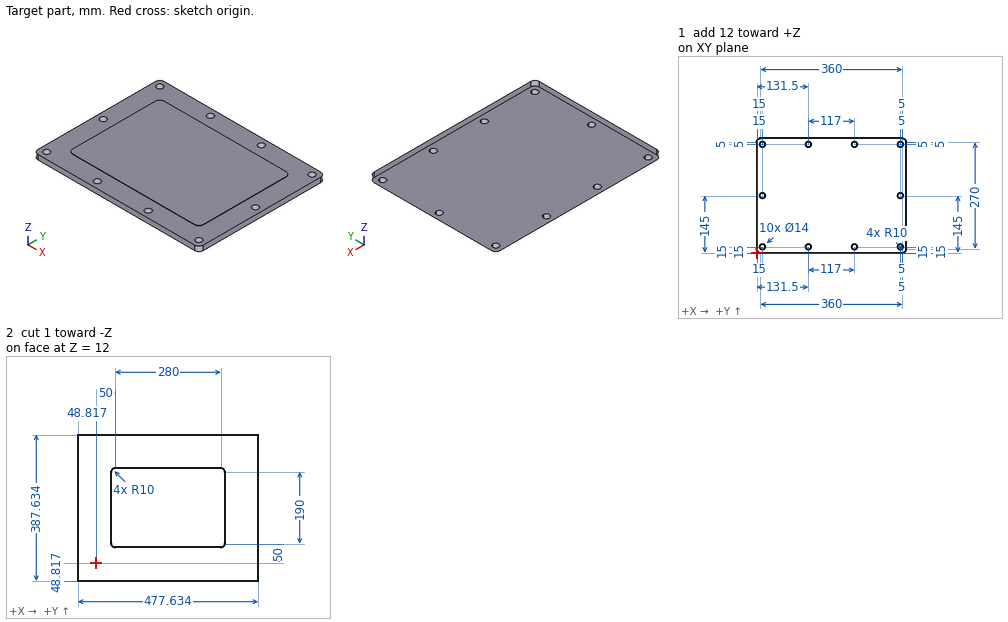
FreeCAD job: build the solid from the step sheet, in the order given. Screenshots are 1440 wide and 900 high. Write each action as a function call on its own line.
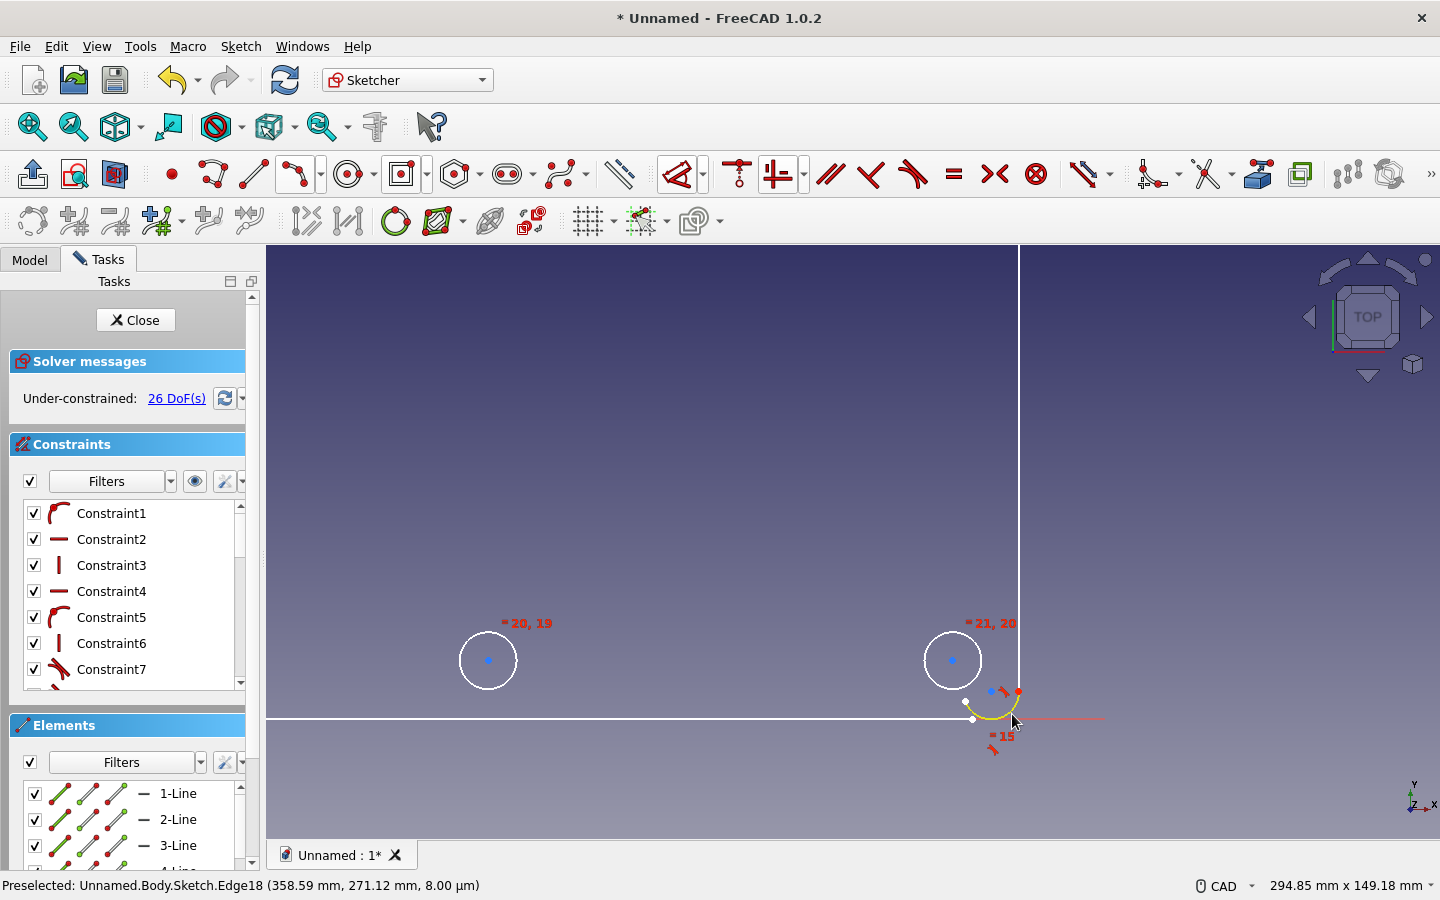
click(1010, 712)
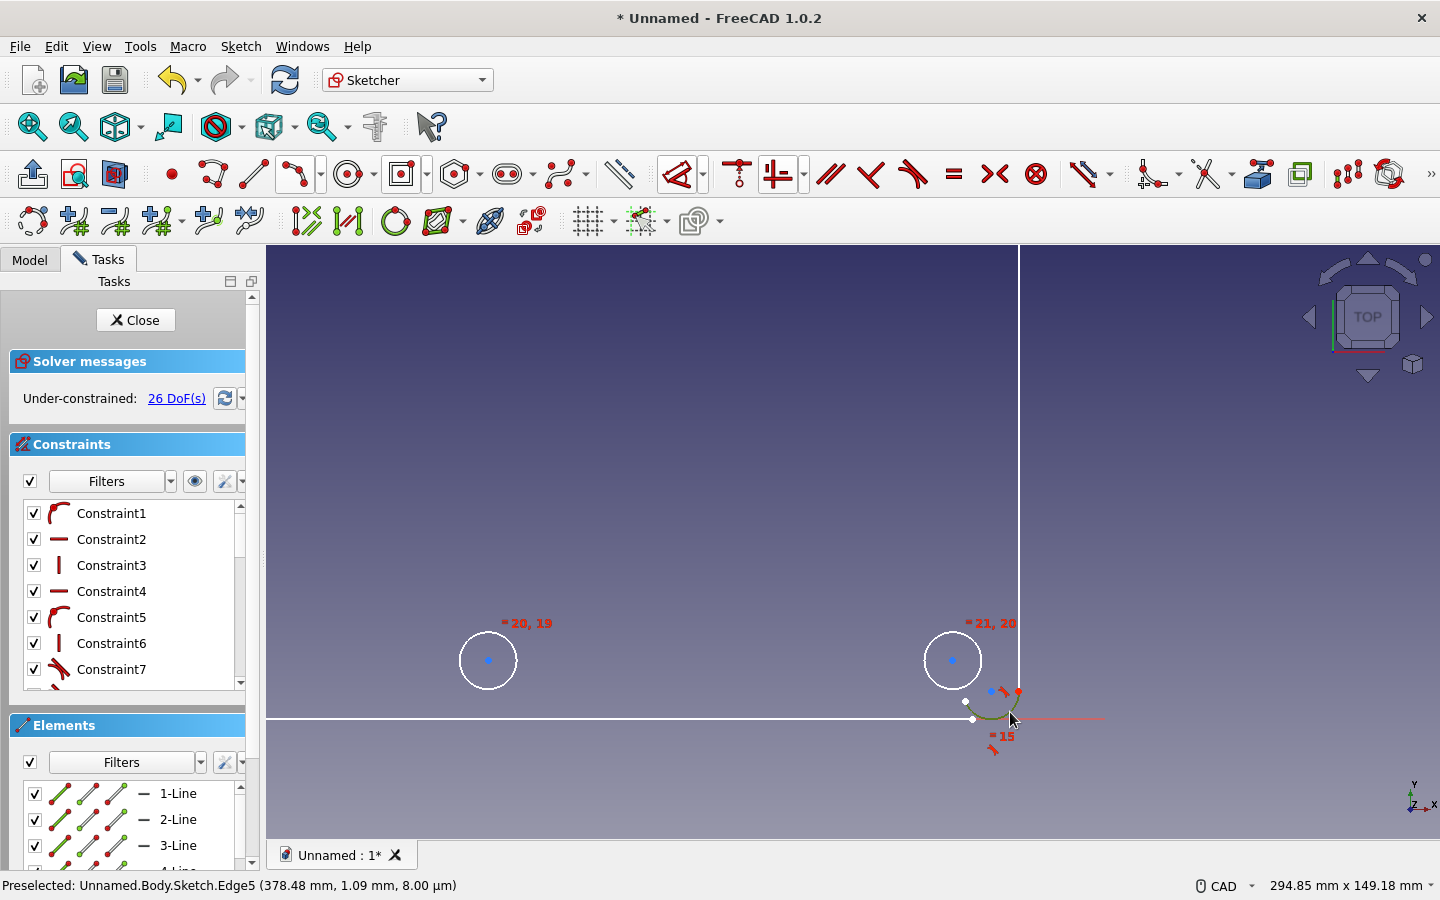
click(702, 174)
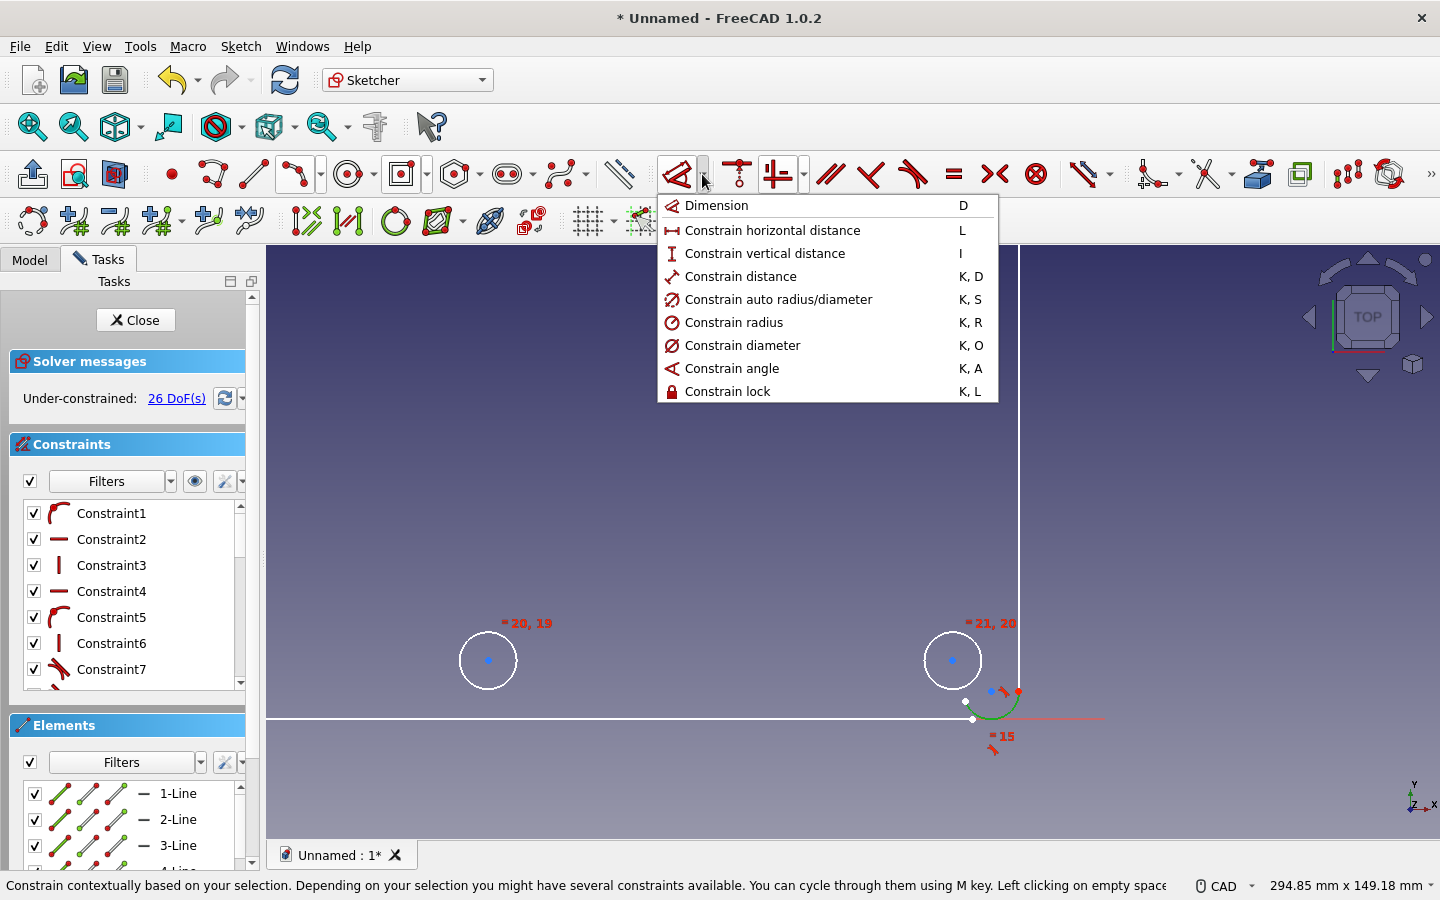
click(828, 322)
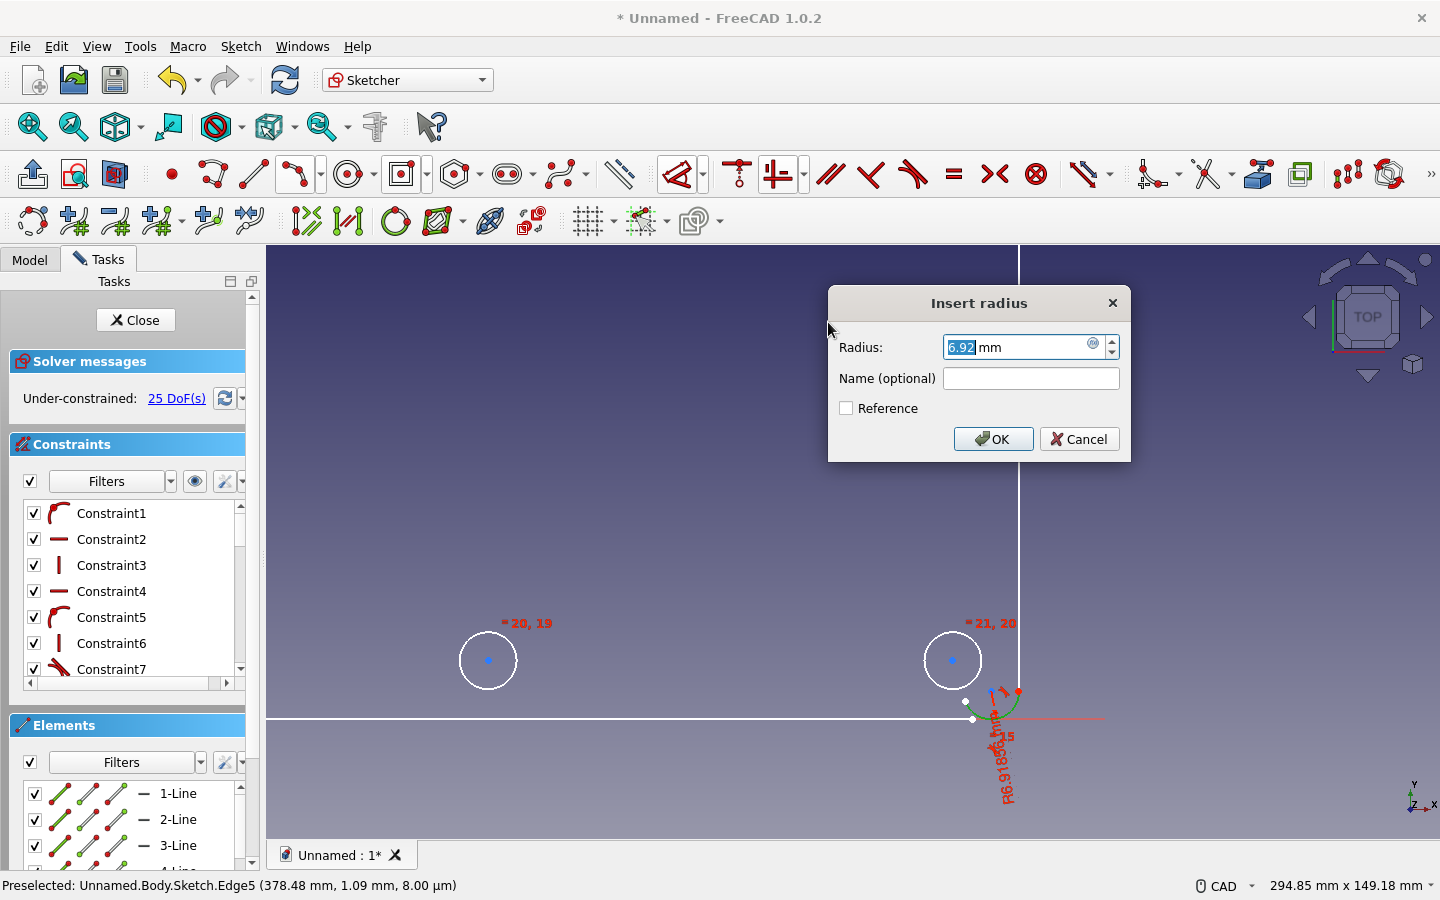
text(10)
key(Return)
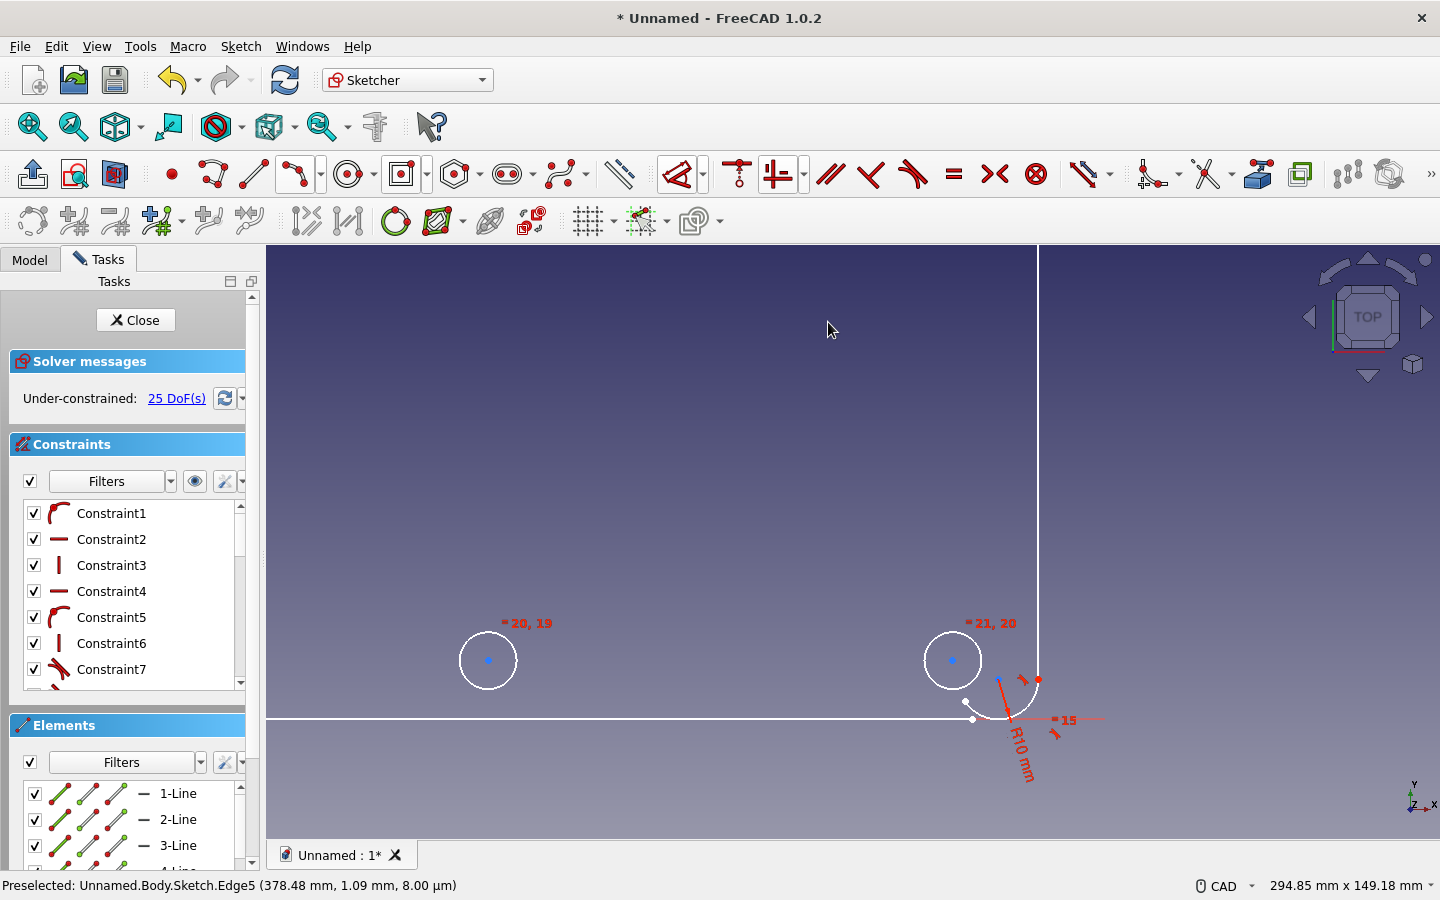
scroll(1012, 714, down, 6)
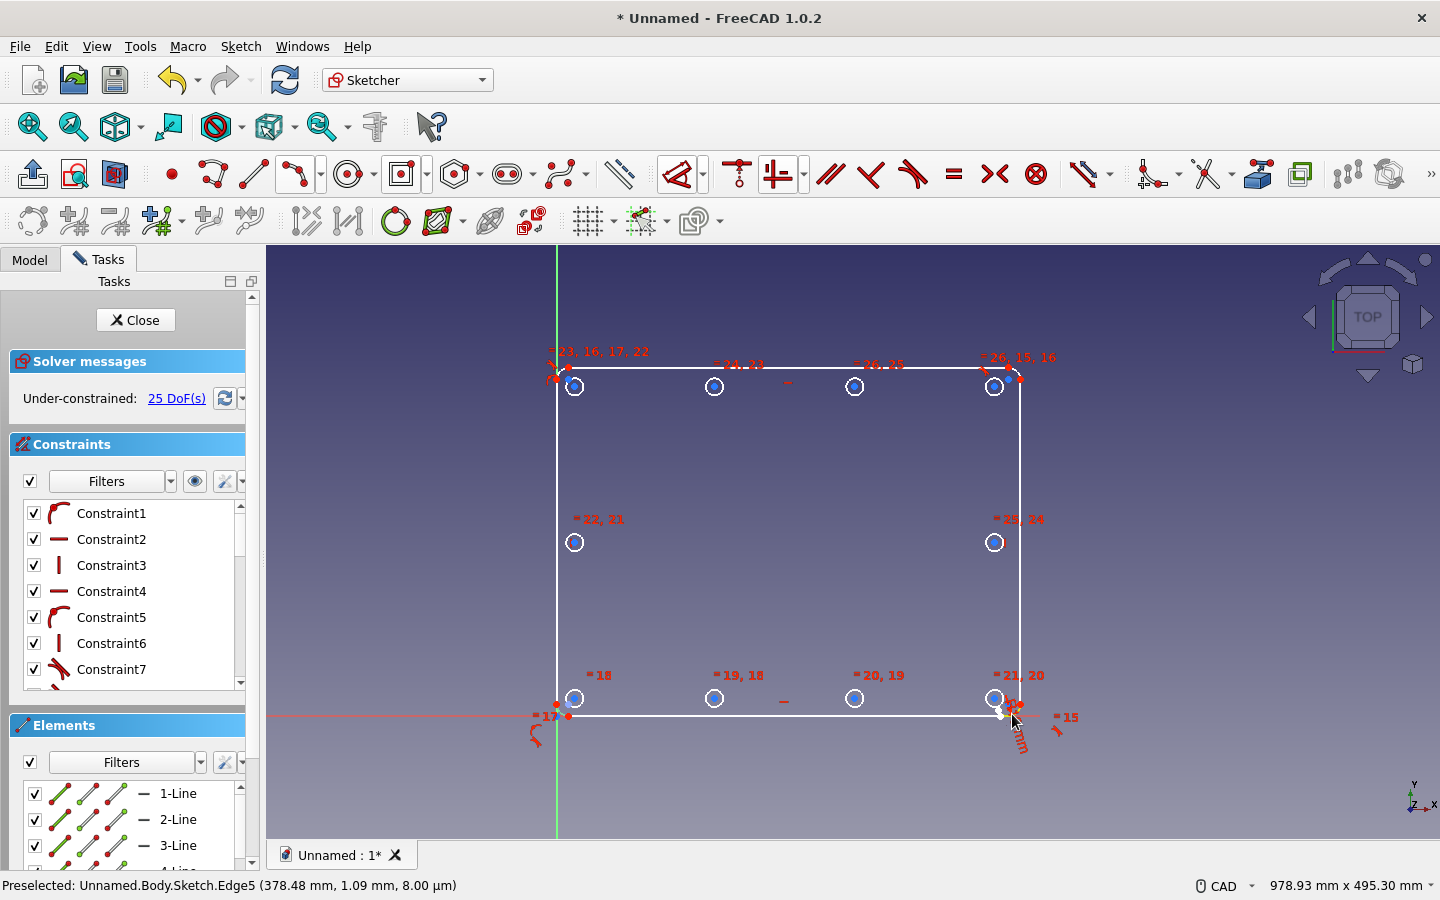
scroll(581, 692, up, 5)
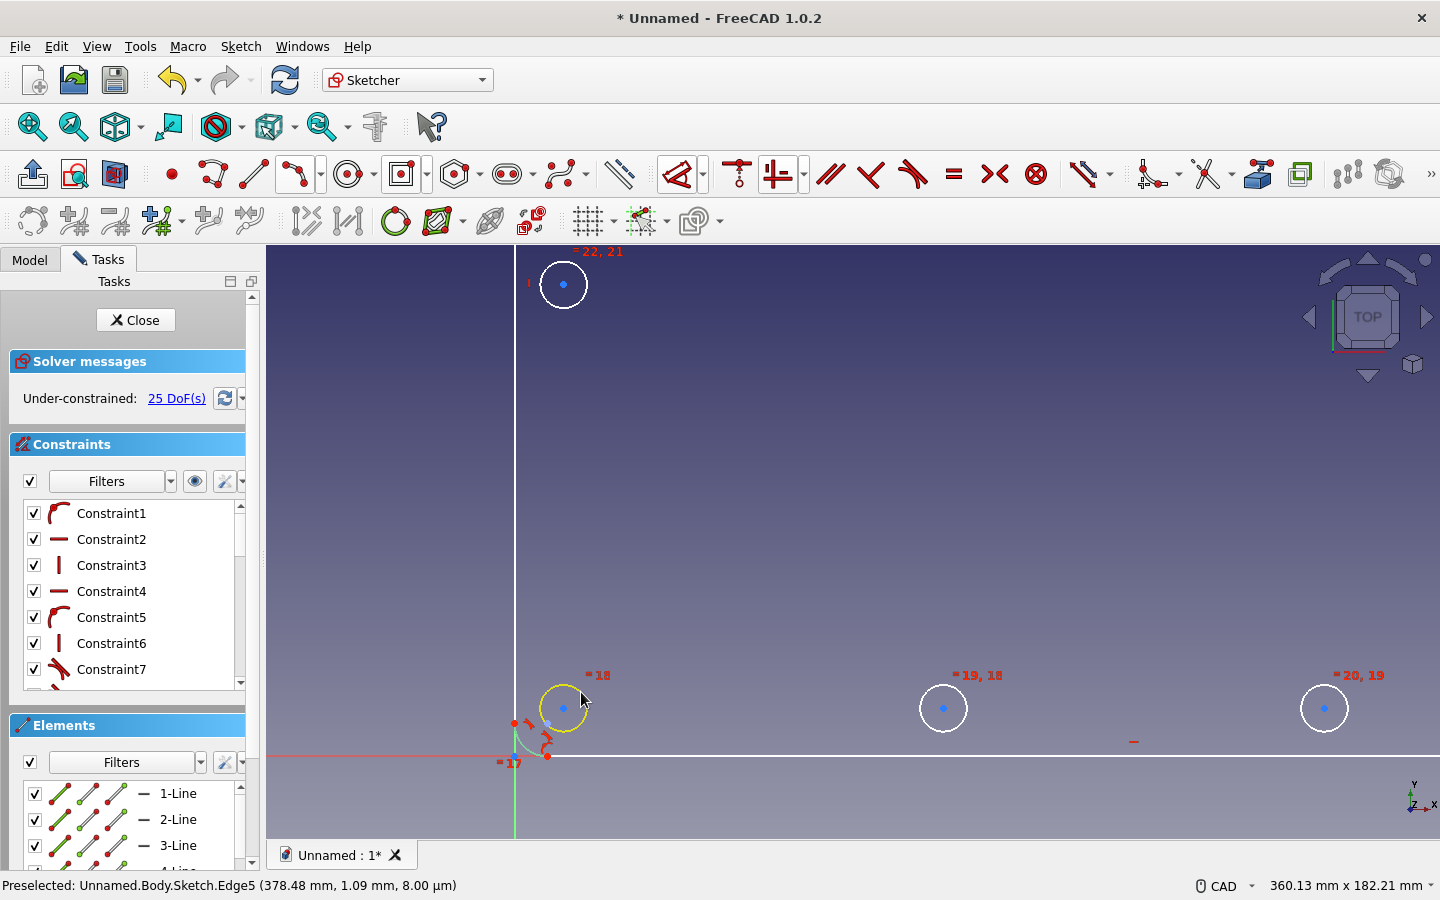
click(580, 692)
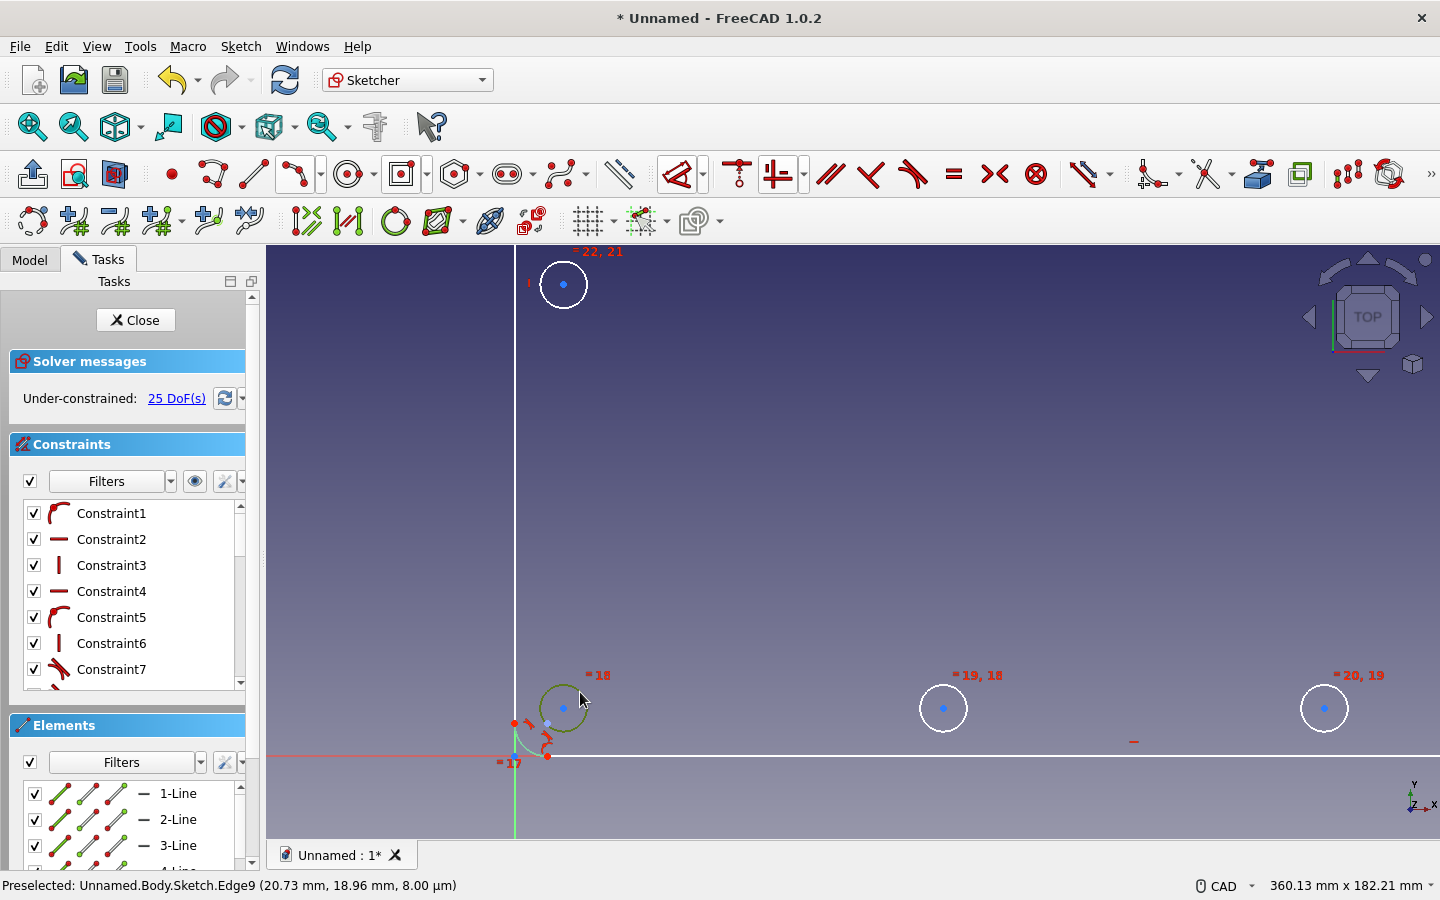
click(702, 174)